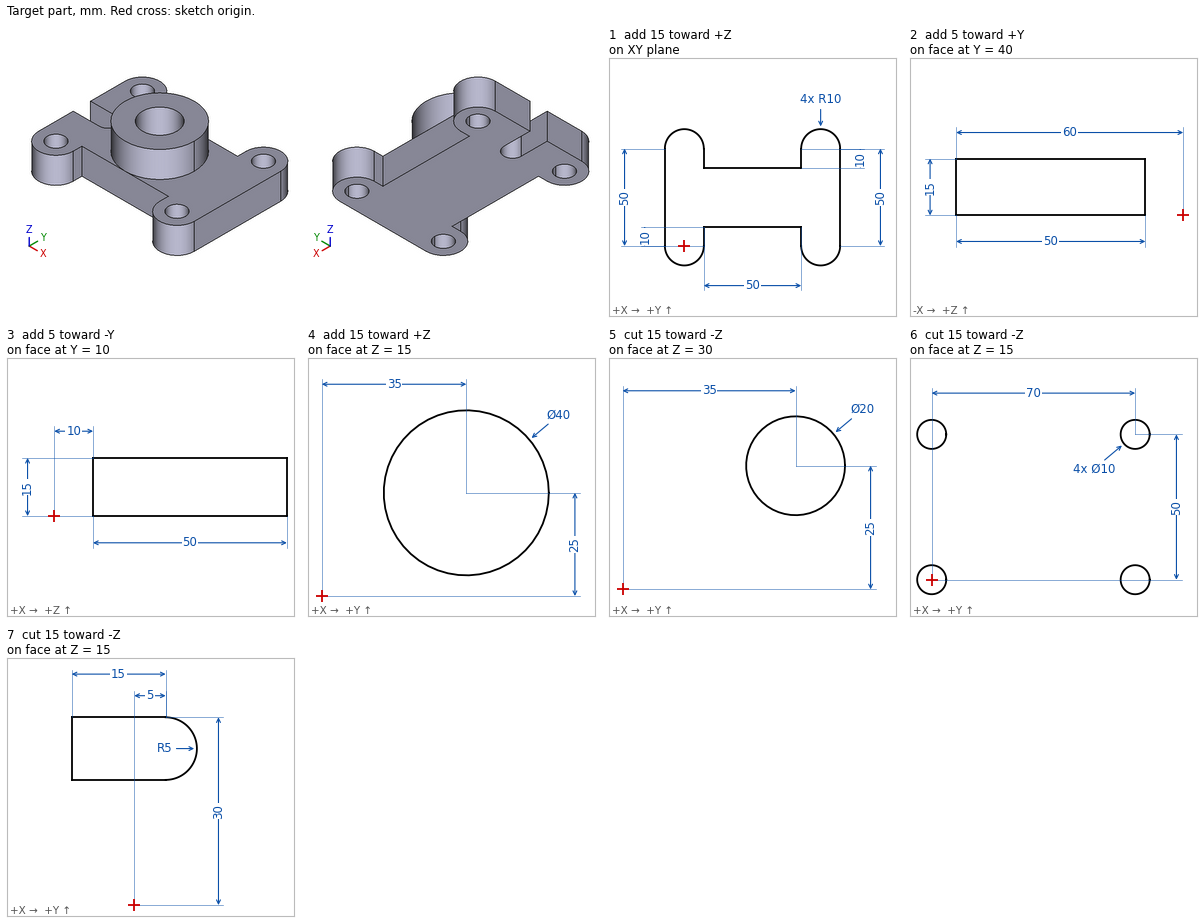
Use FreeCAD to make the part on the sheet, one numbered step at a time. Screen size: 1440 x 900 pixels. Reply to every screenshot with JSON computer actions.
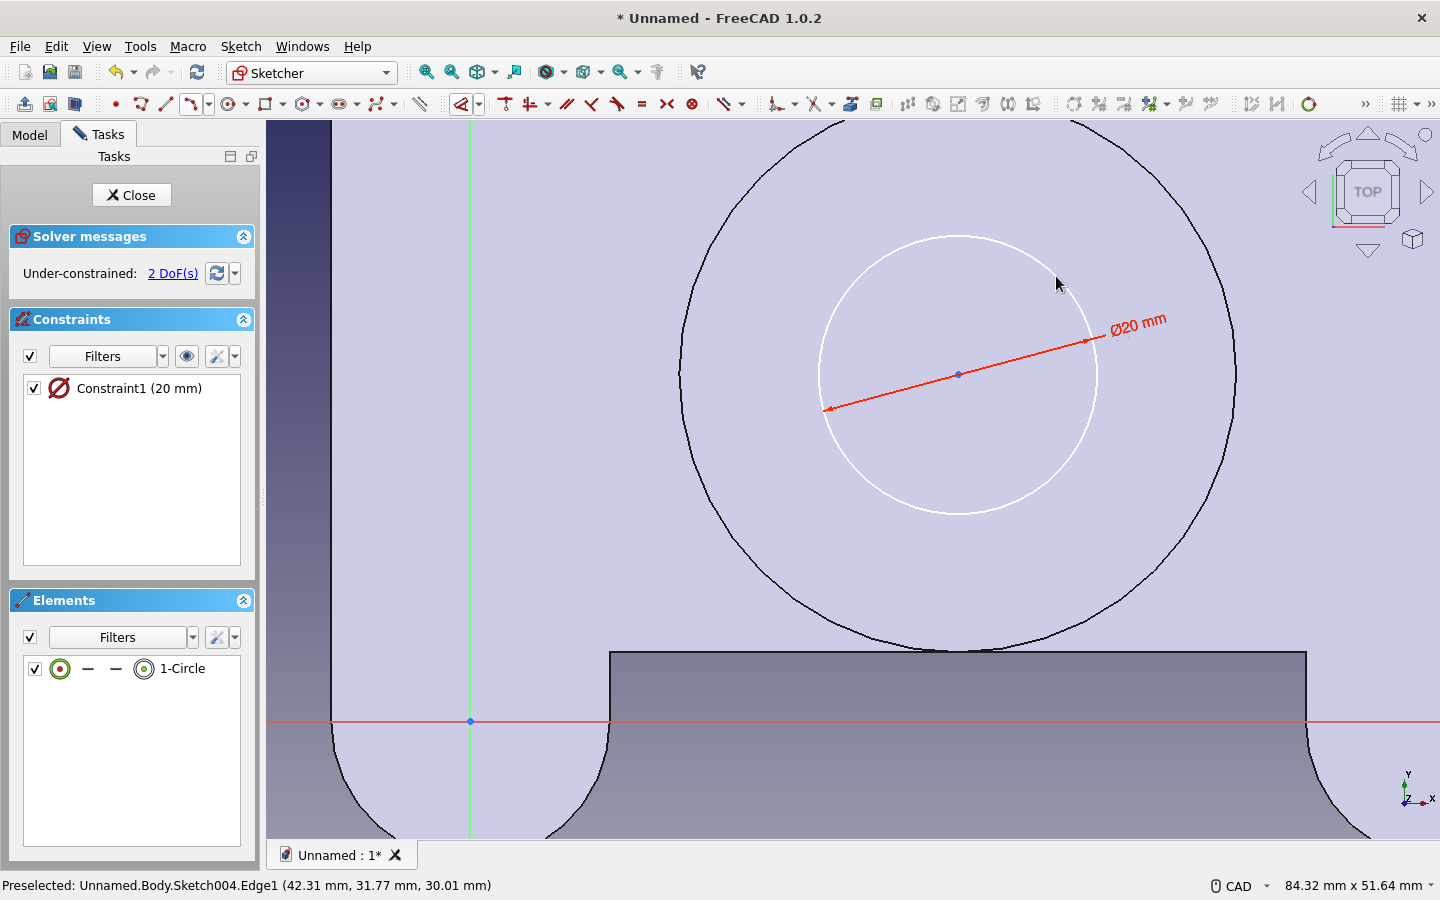
{"action": "left_click", "coordinate": [958, 375]}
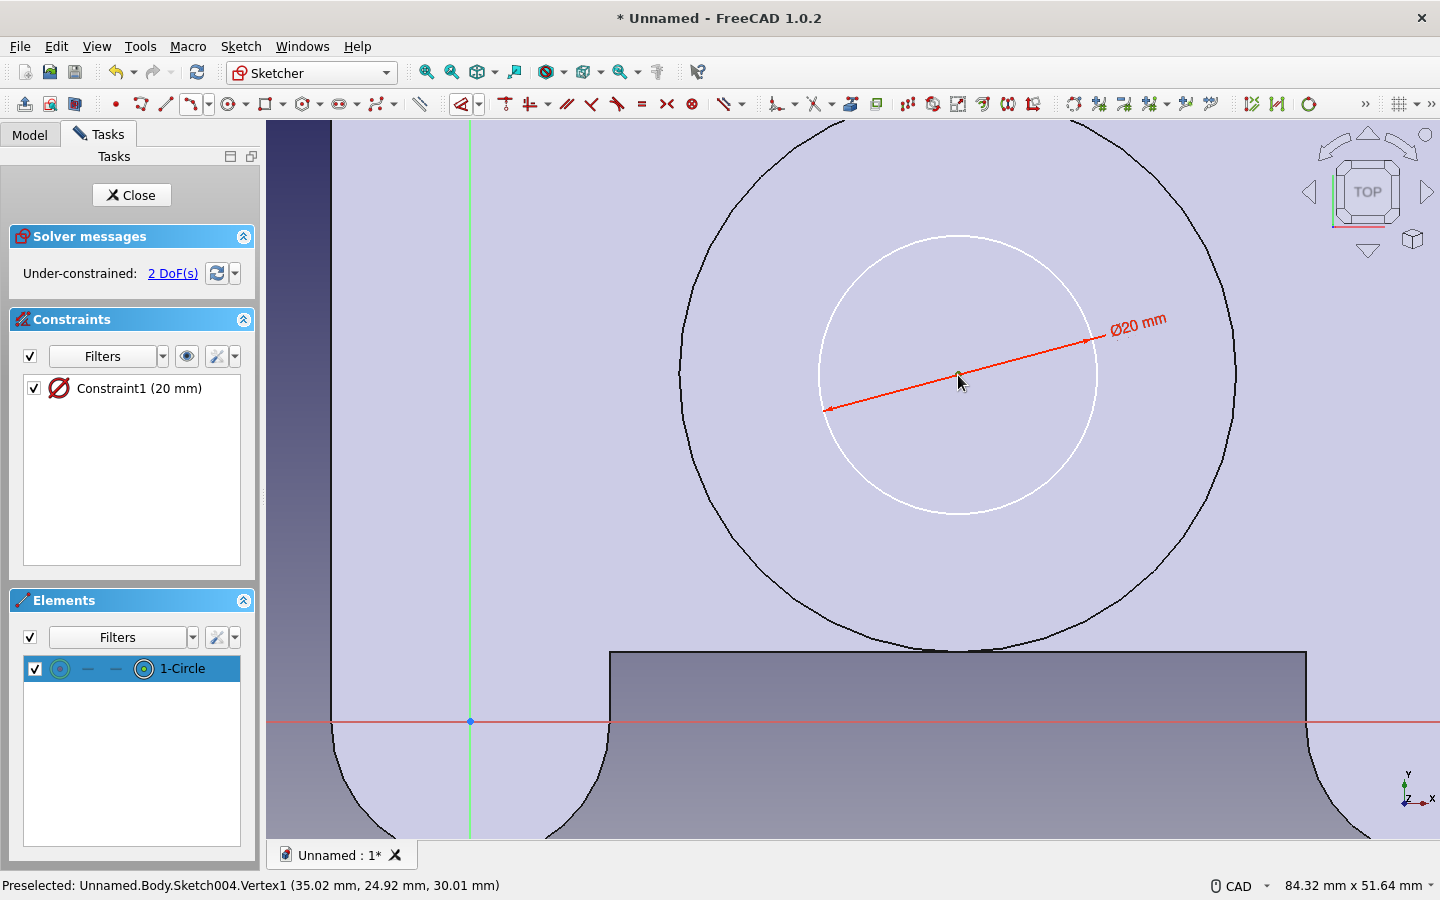
{"action": "key", "text": "l"}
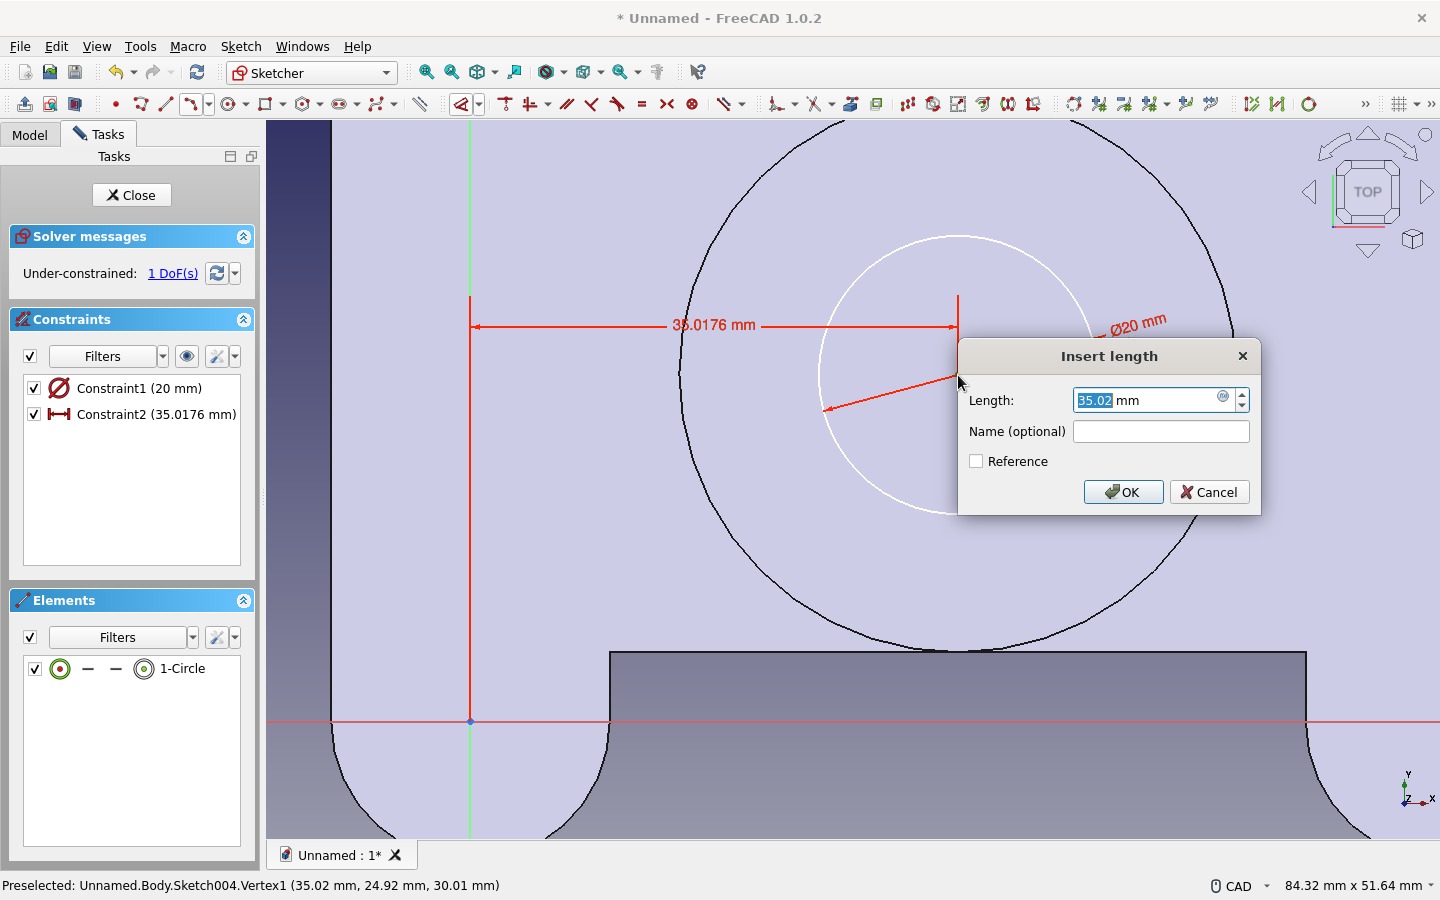
{"action": "type", "text": "35"}
{"action": "key", "text": "Return"}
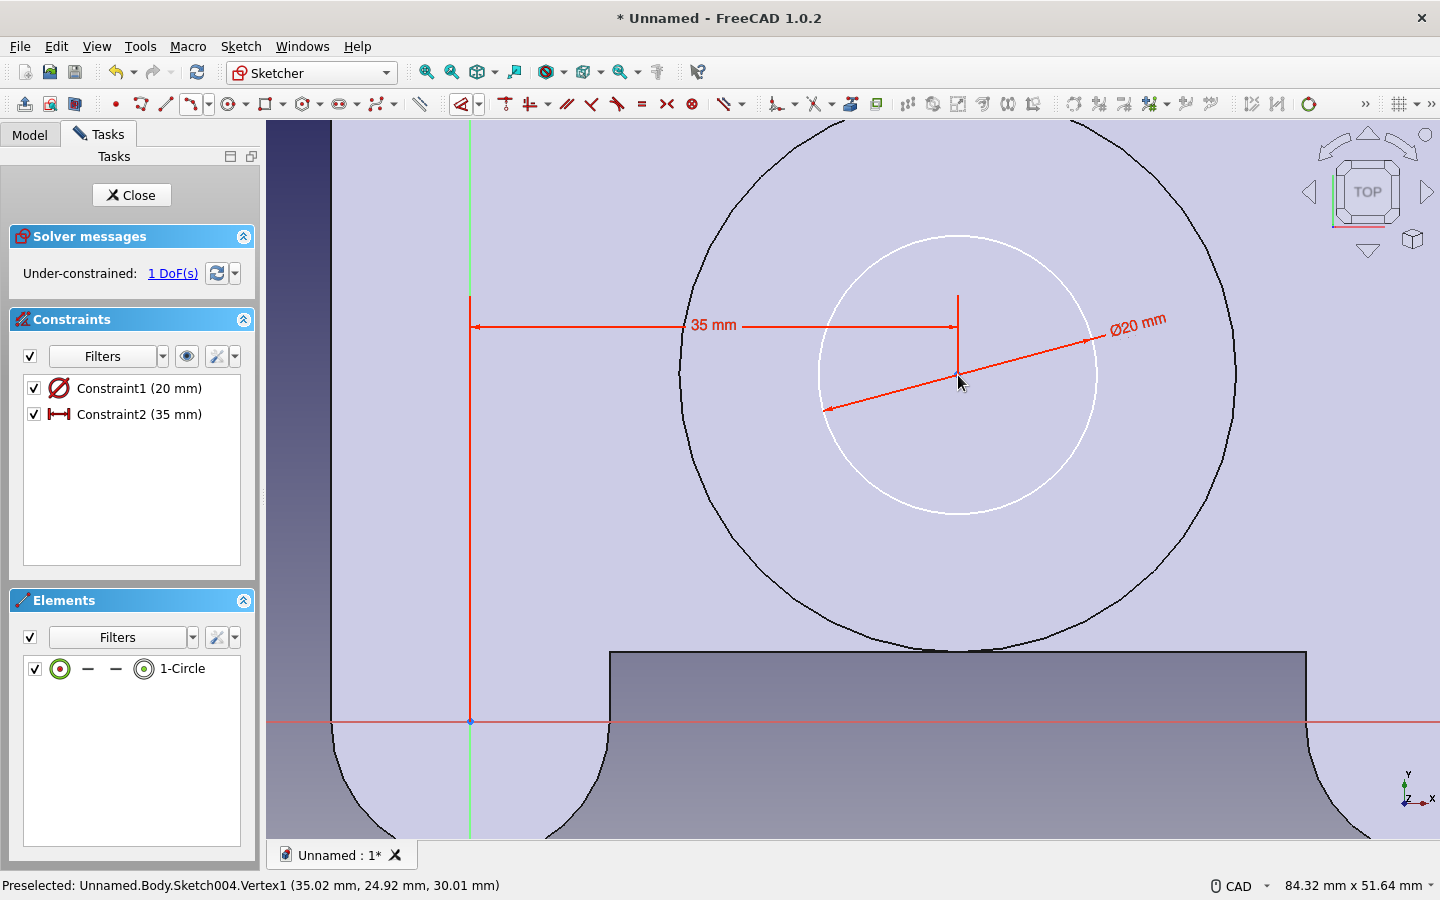
{"action": "left_click", "coordinate": [958, 375]}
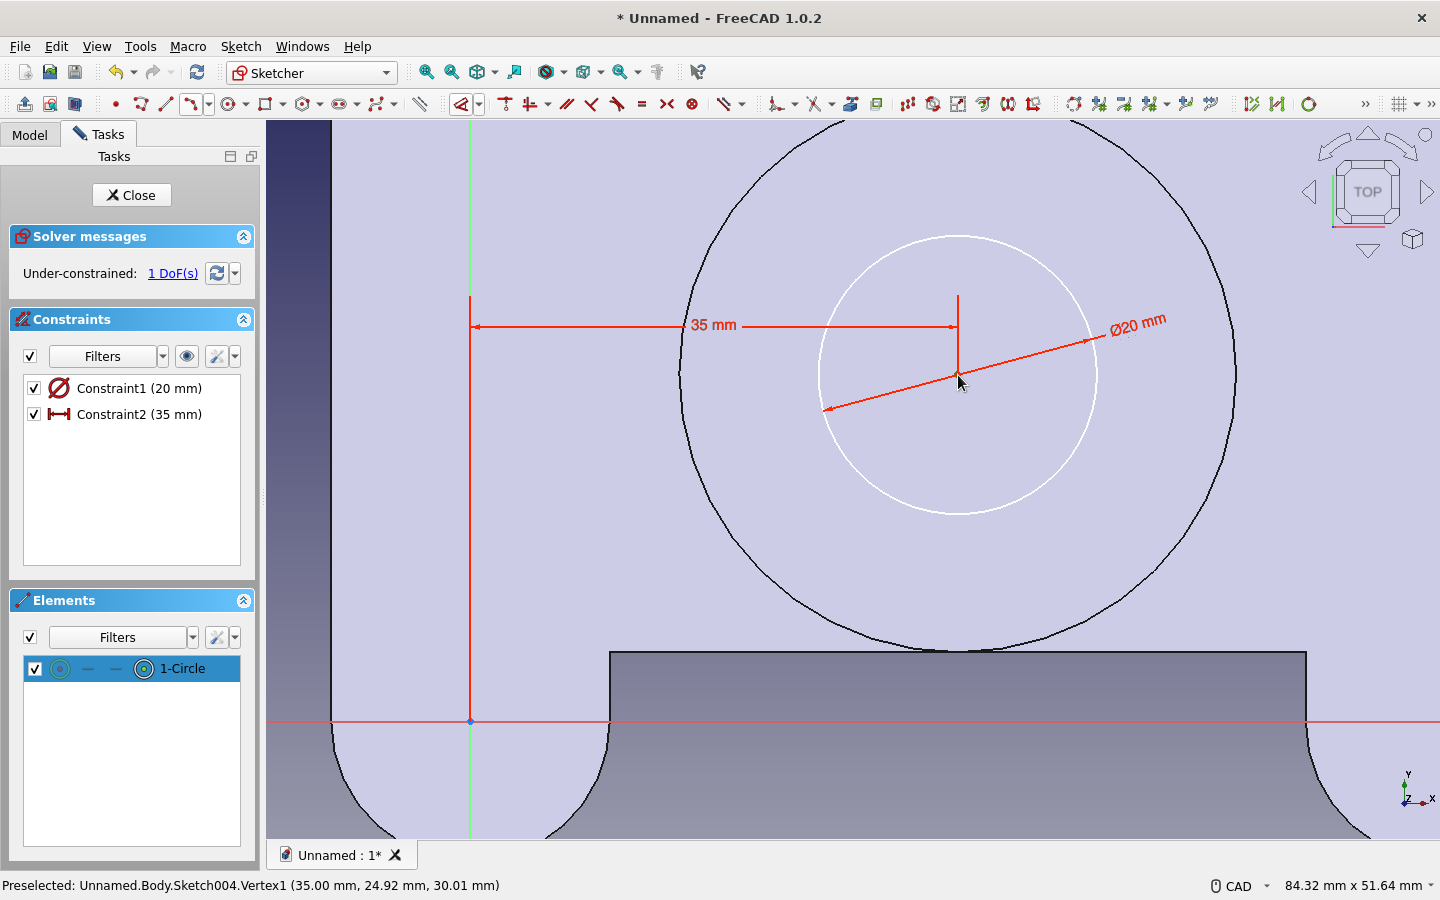
{"action": "left_click", "coordinate": [478, 104]}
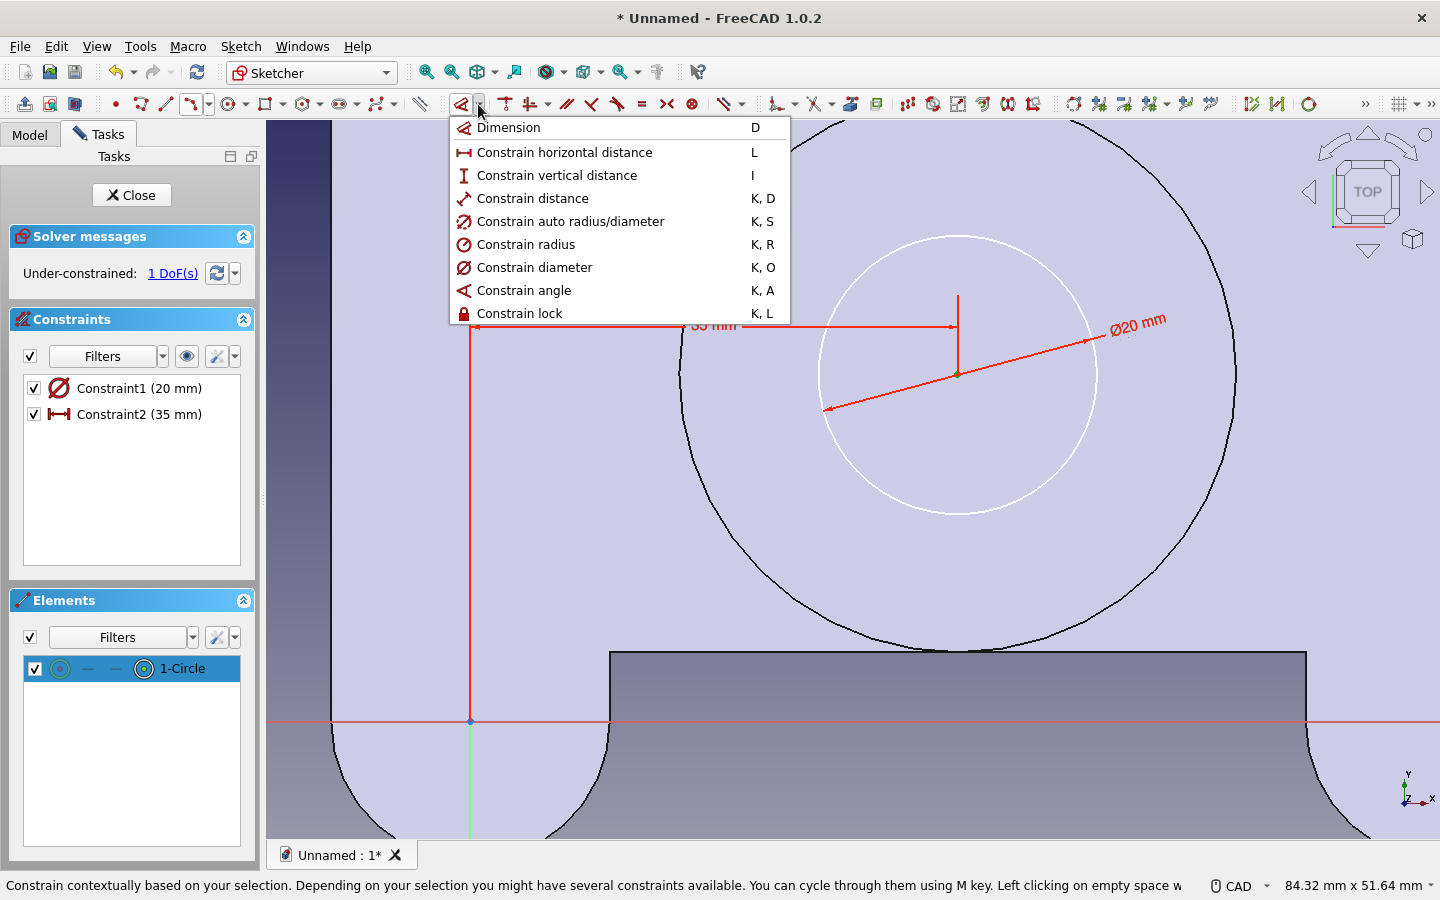
{"action": "left_click", "coordinate": [620, 176]}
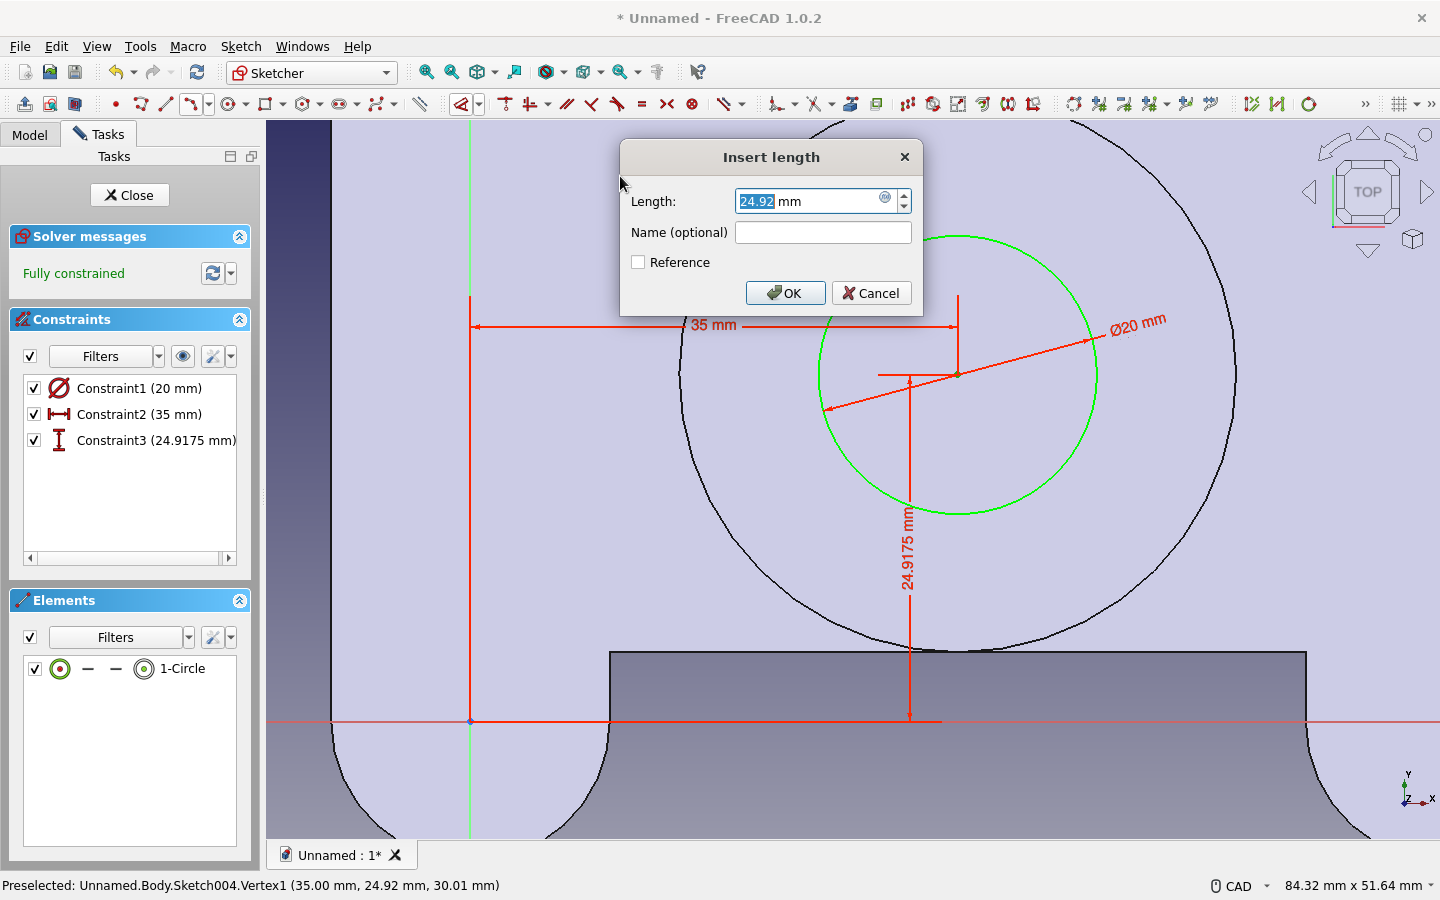
{"action": "type", "text": "25"}
{"action": "key", "text": "Return"}